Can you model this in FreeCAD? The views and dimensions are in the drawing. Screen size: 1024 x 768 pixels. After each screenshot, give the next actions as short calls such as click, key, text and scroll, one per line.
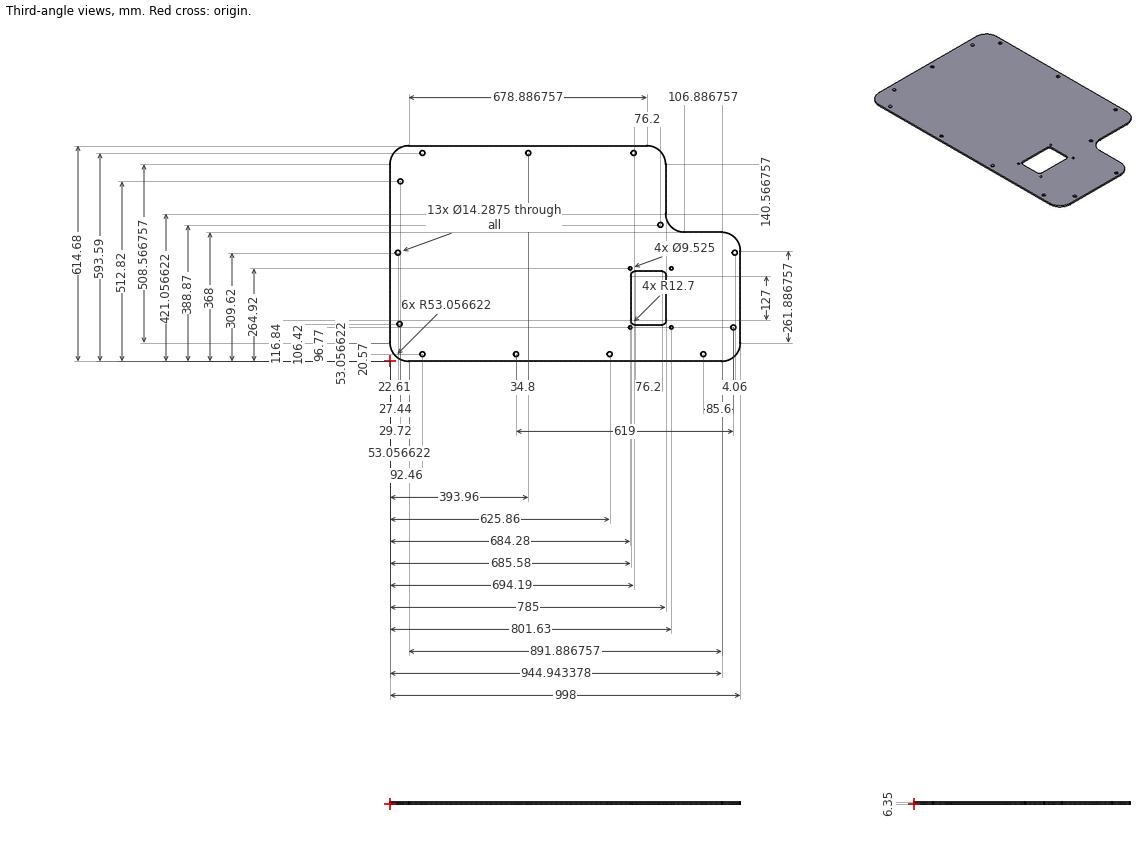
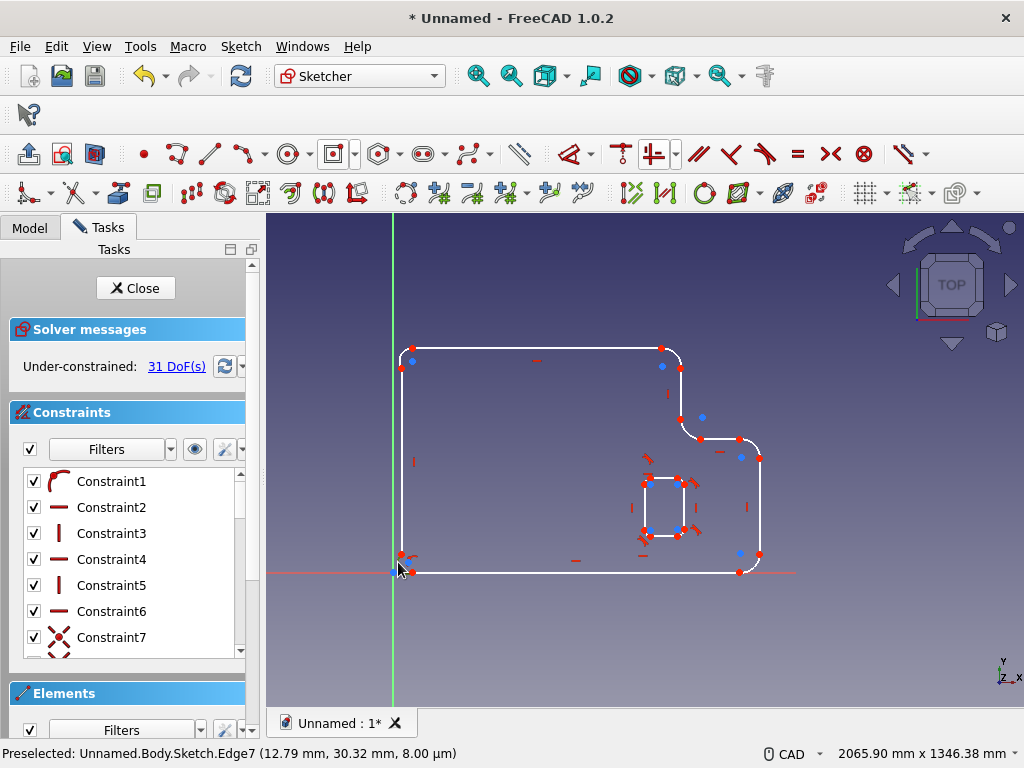
scroll(757, 563, up, 3)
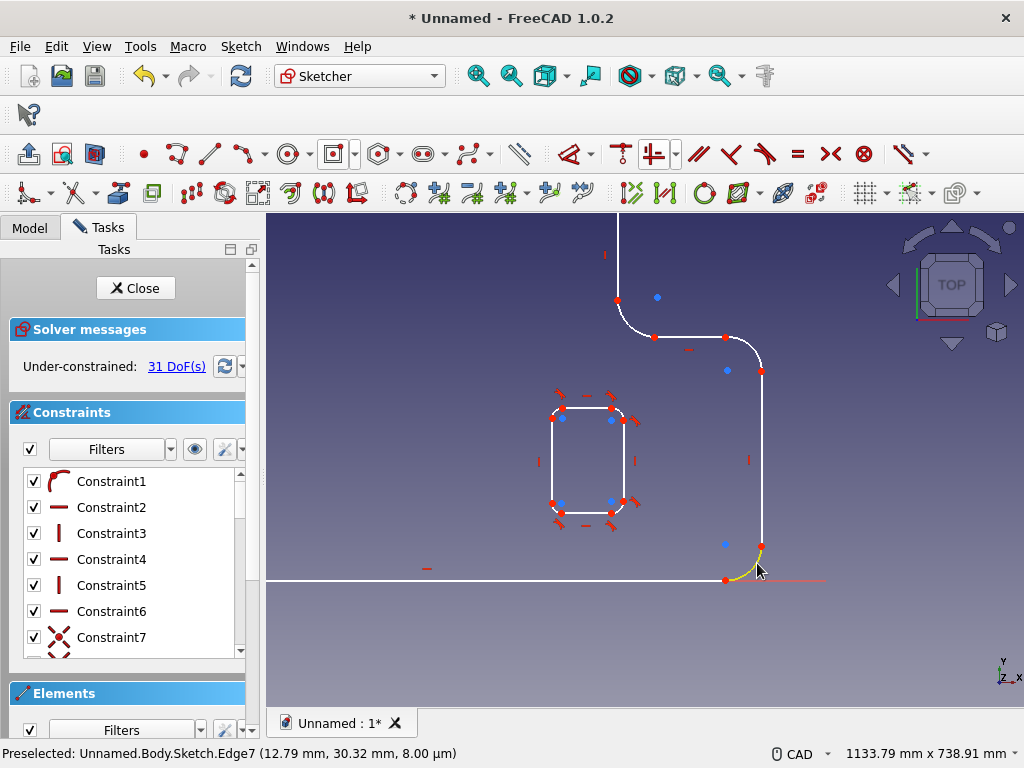
click(757, 562)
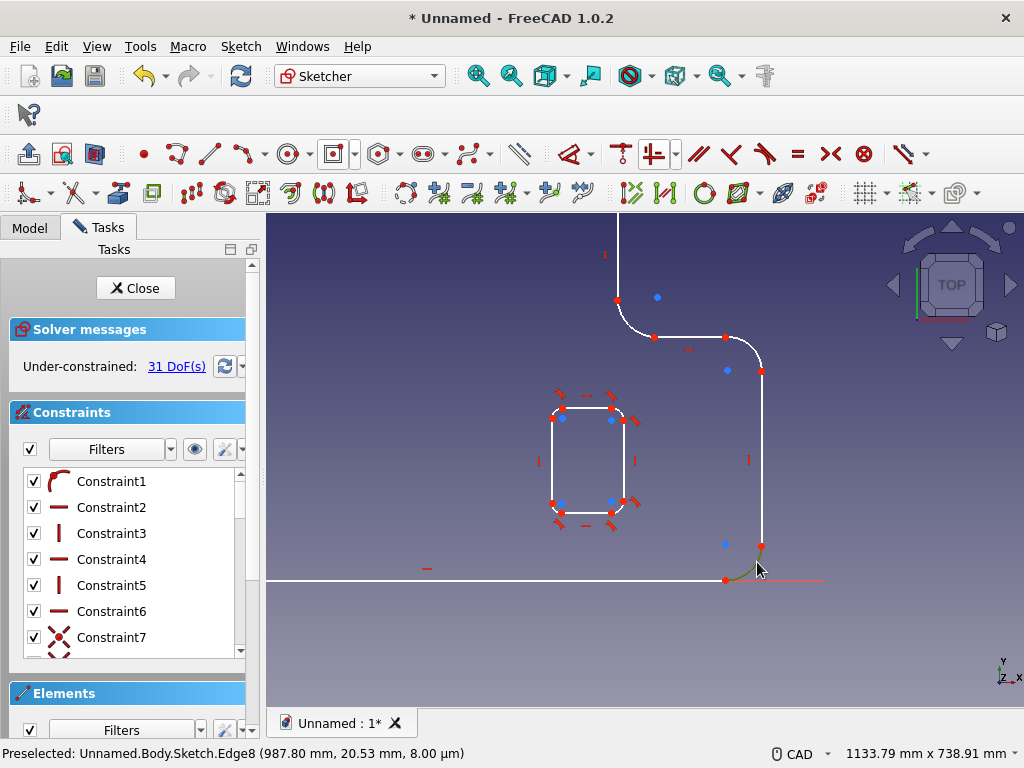
click(758, 355)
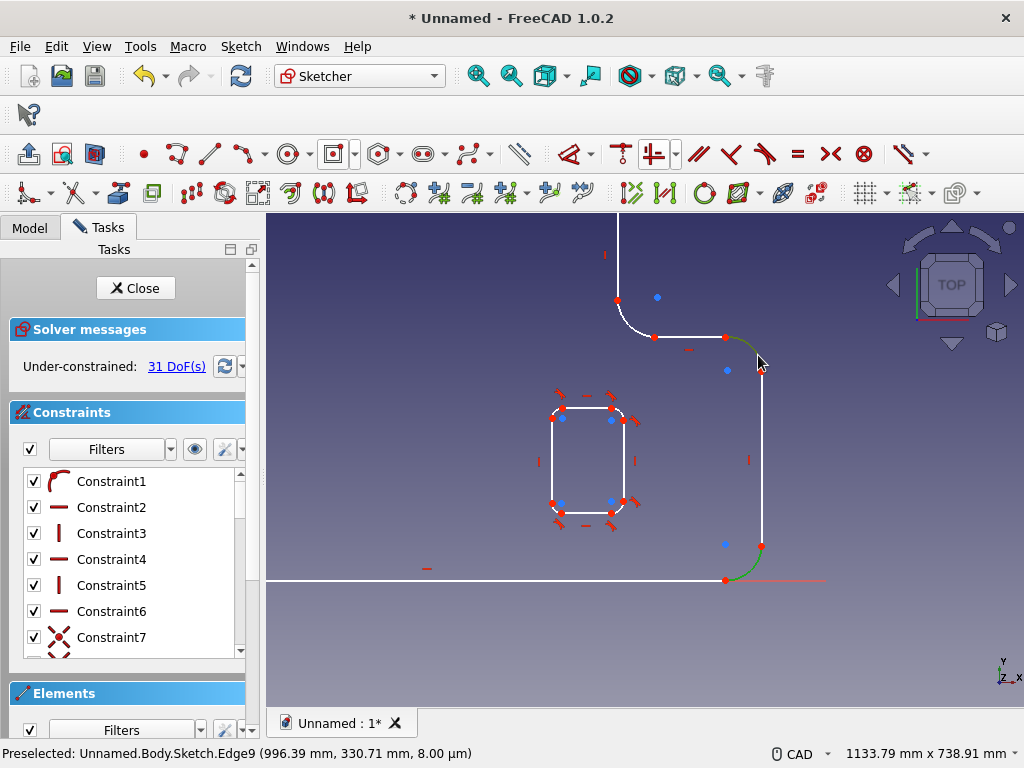
click(623, 317)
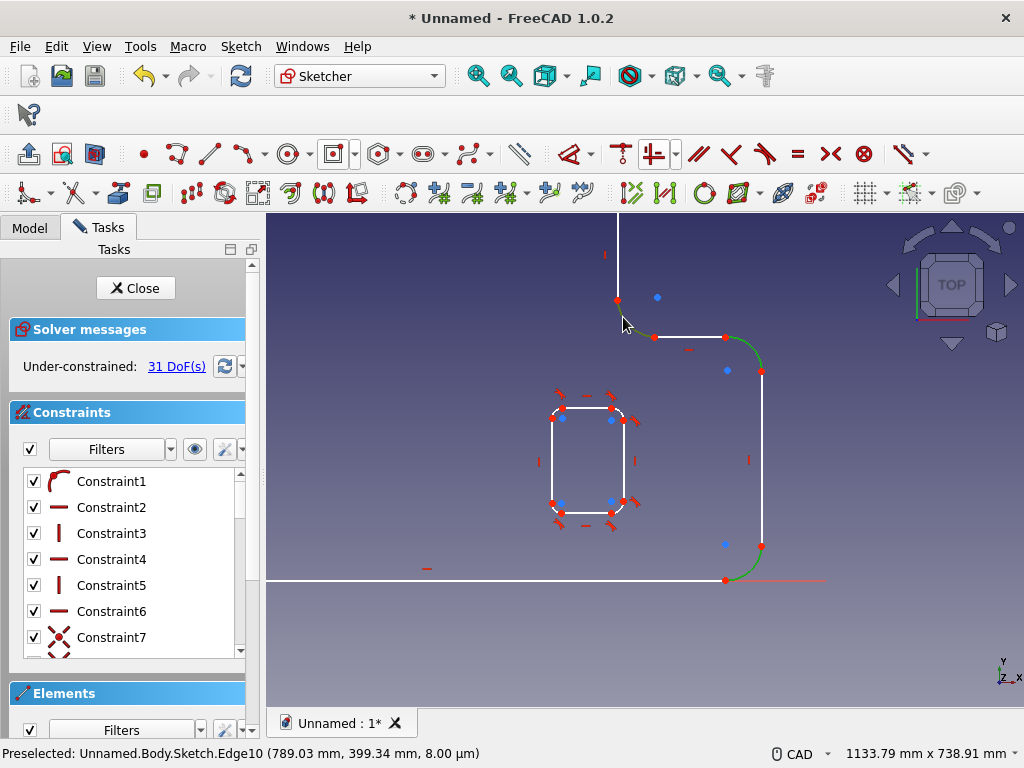
scroll(758, 563, down, 3)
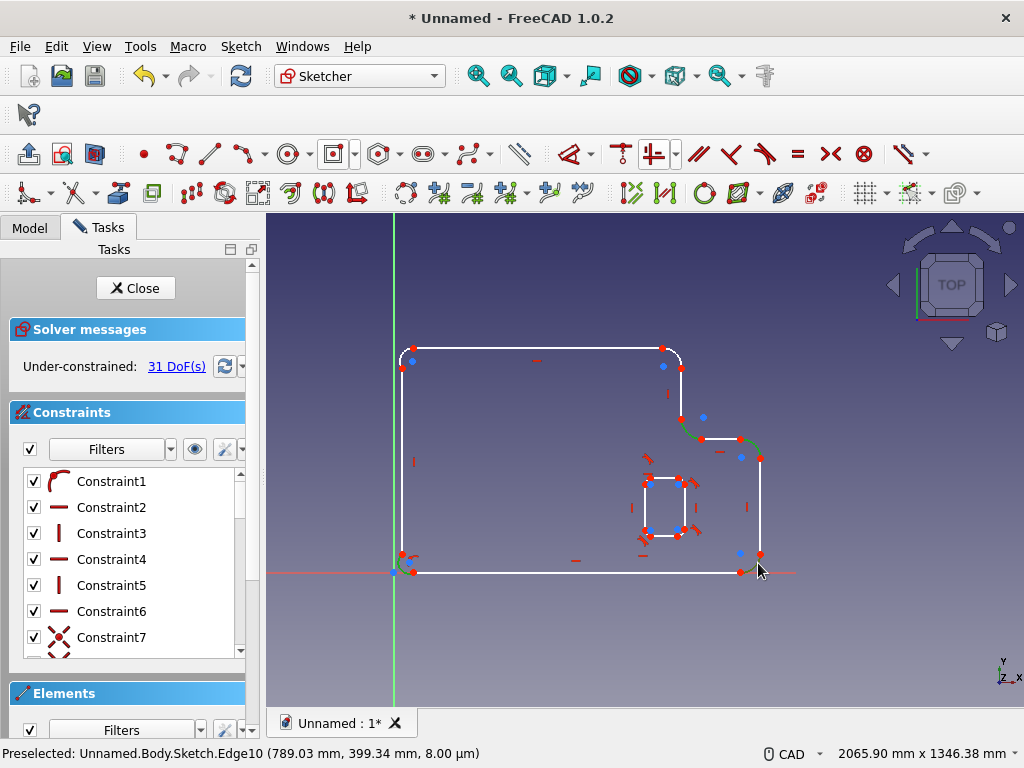
scroll(680, 359, up, 2)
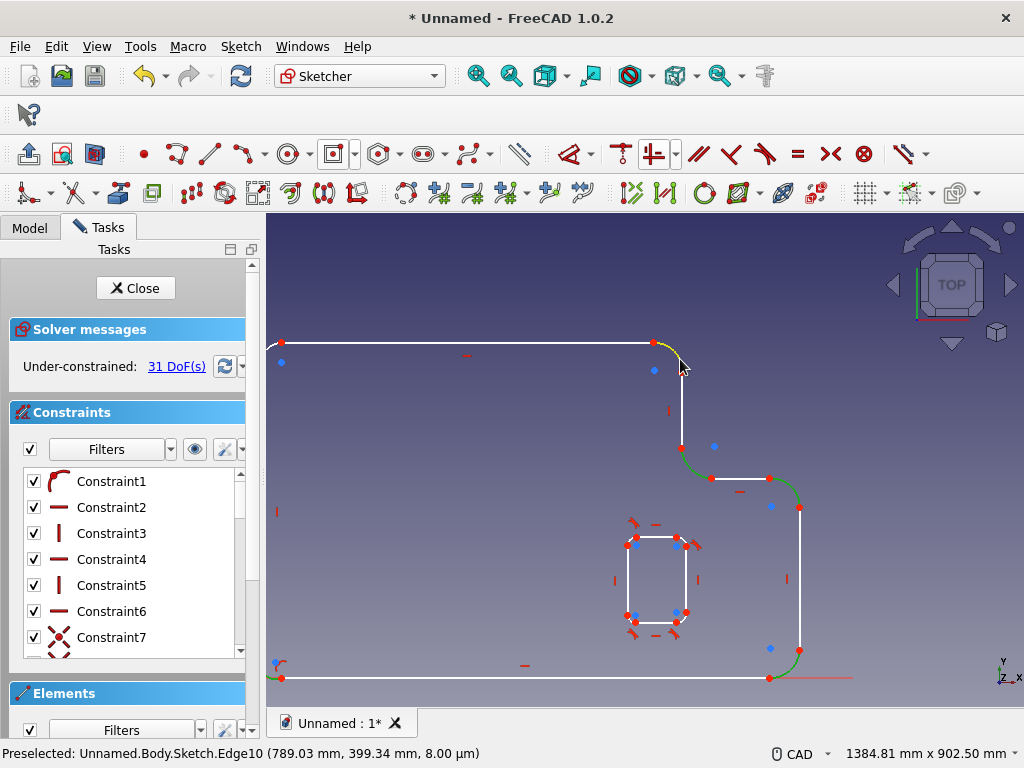
click(680, 359)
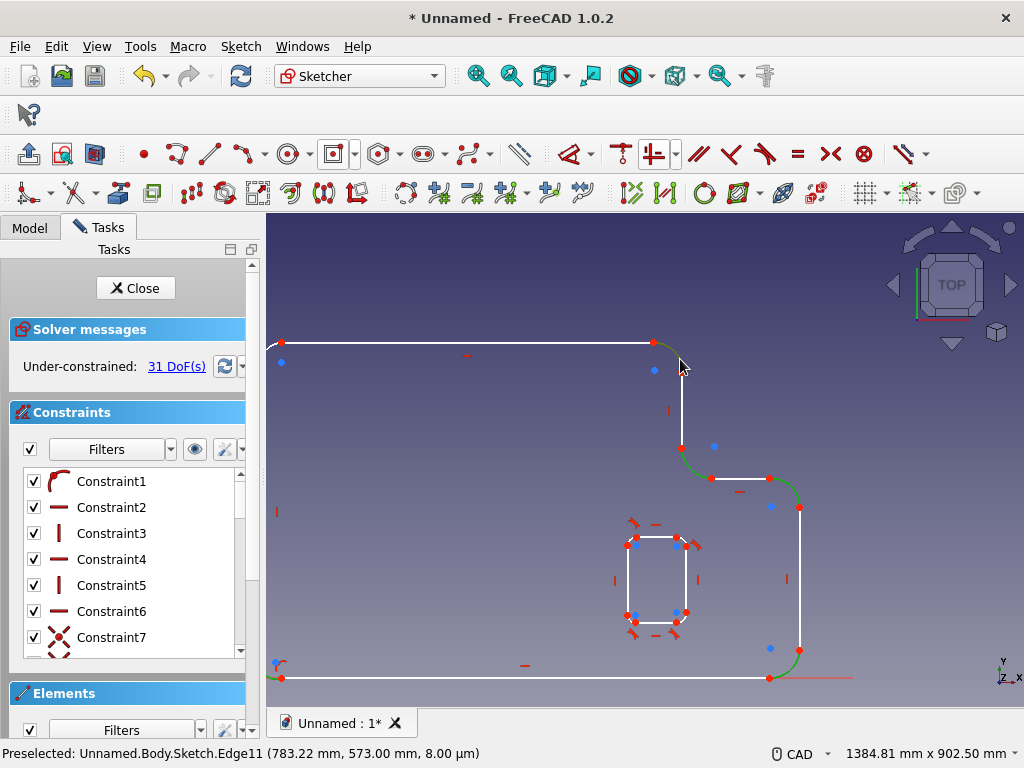
scroll(680, 359, down, 2)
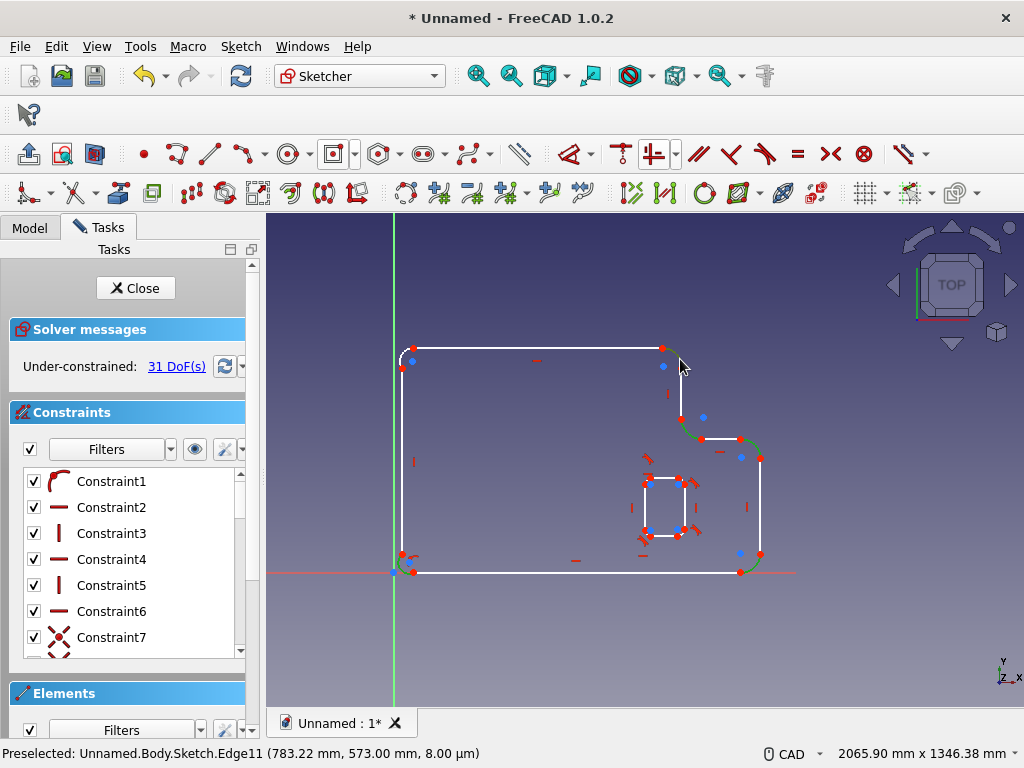
scroll(405, 351, up, 3)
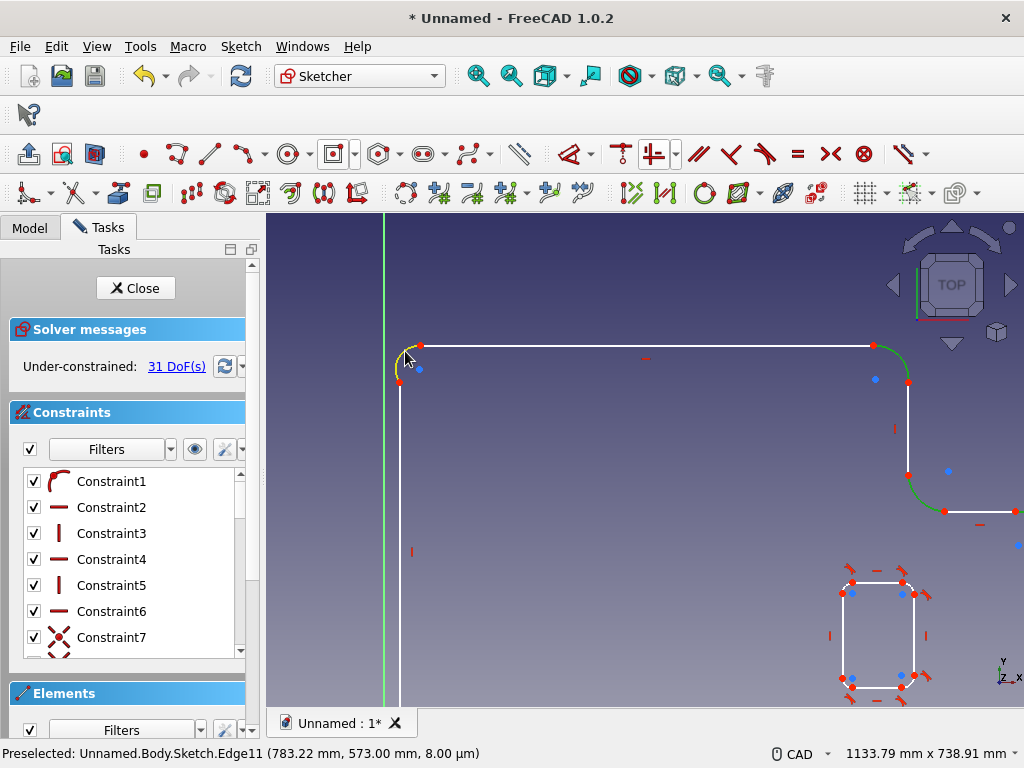
click(405, 350)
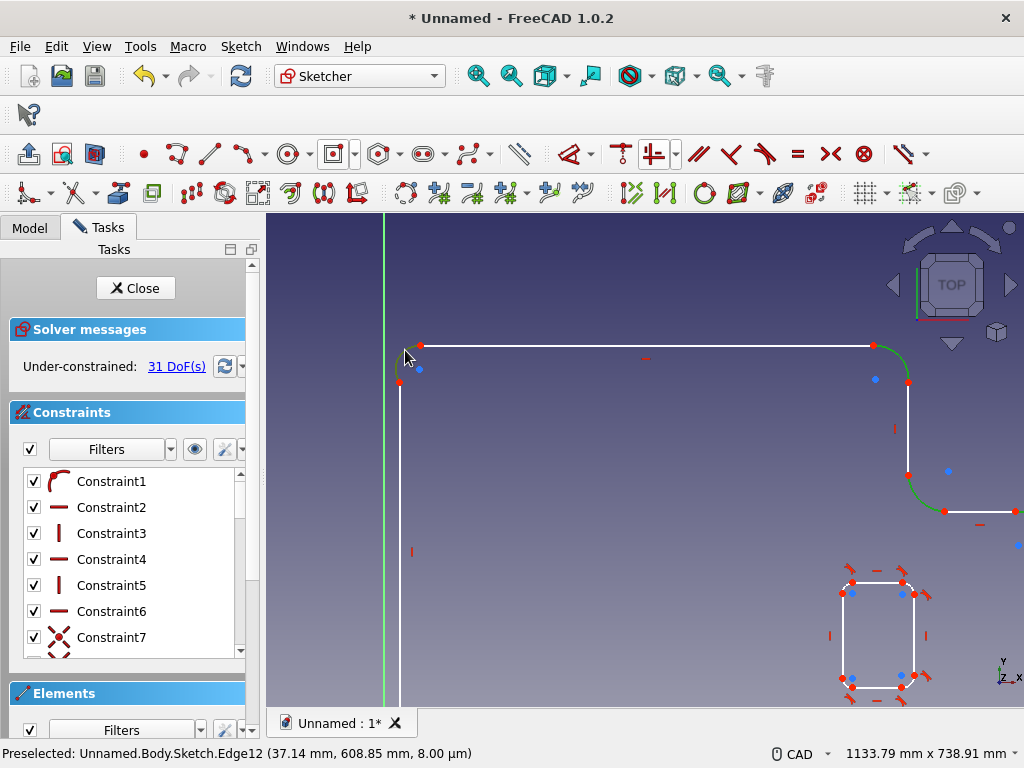
click(798, 154)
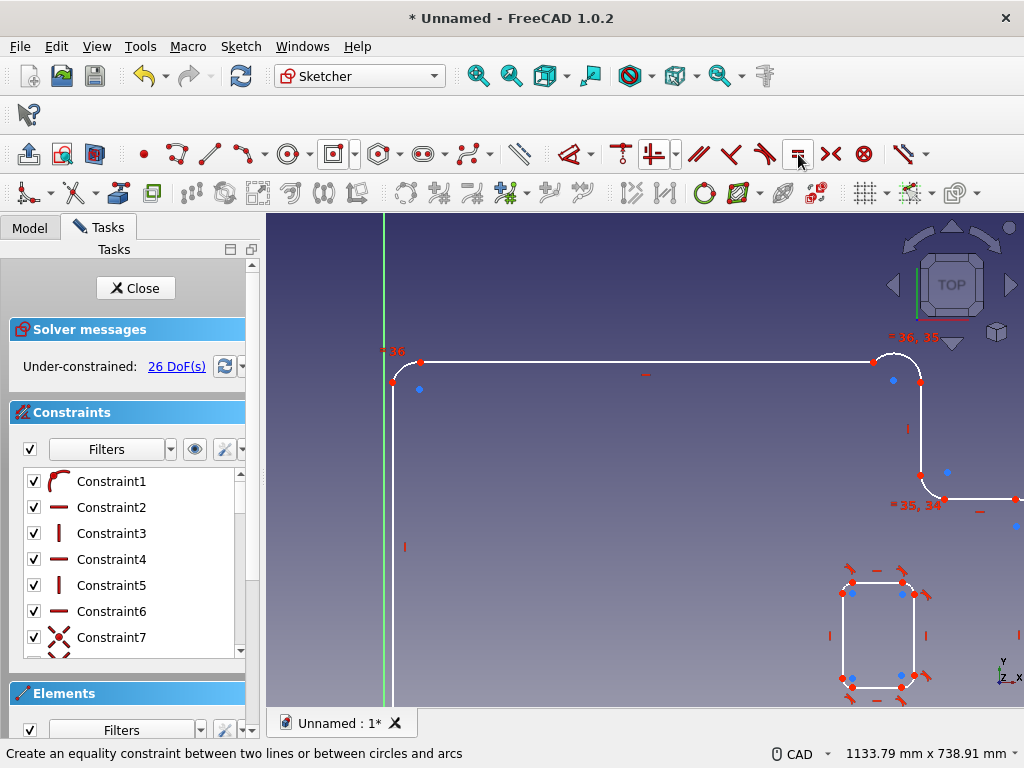
scroll(846, 586, up, 3)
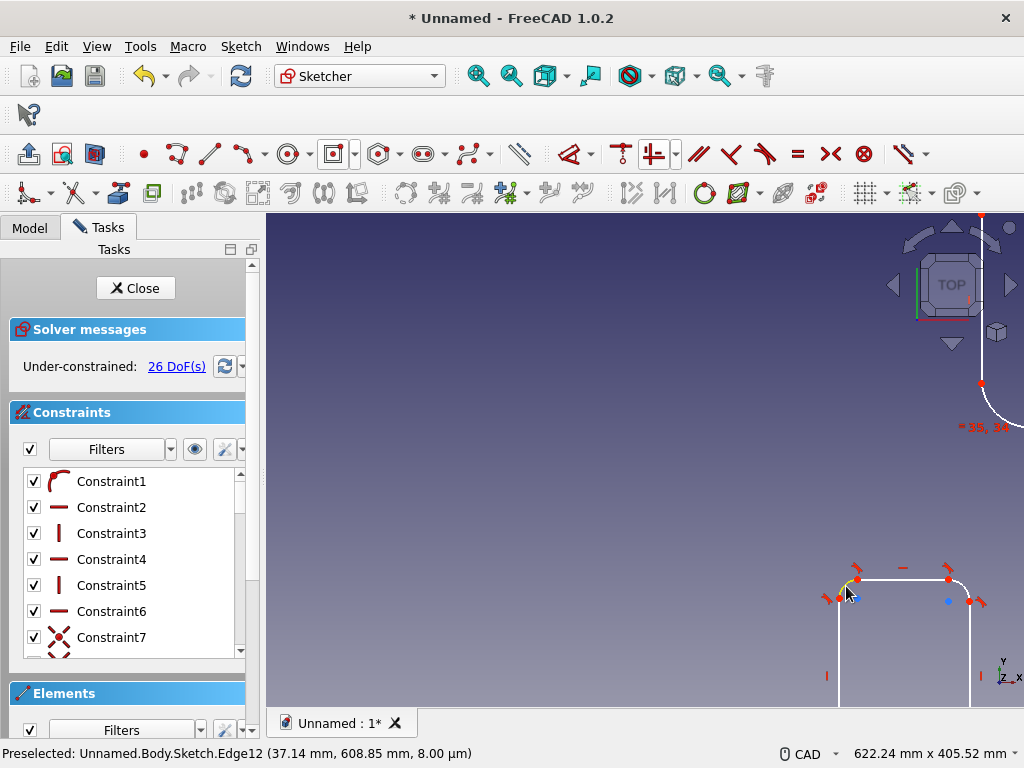
click(845, 585)